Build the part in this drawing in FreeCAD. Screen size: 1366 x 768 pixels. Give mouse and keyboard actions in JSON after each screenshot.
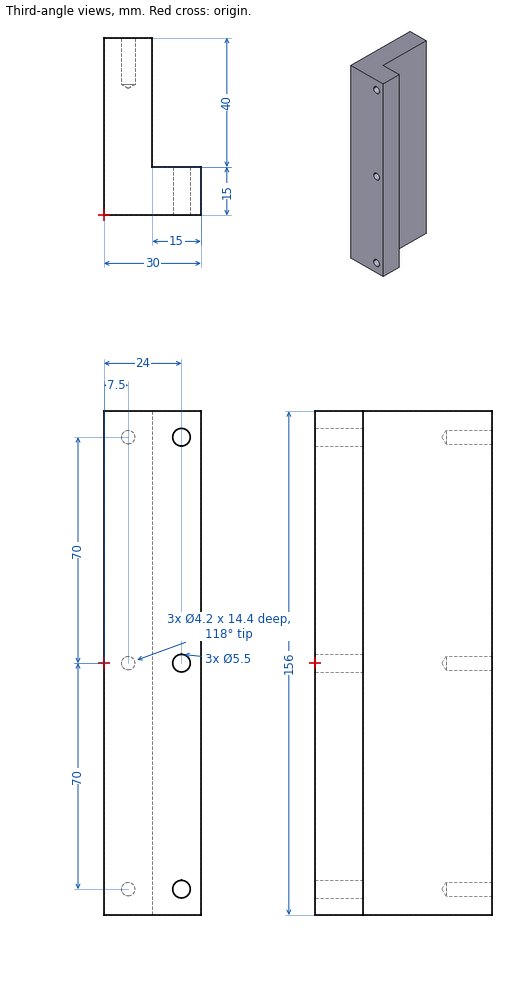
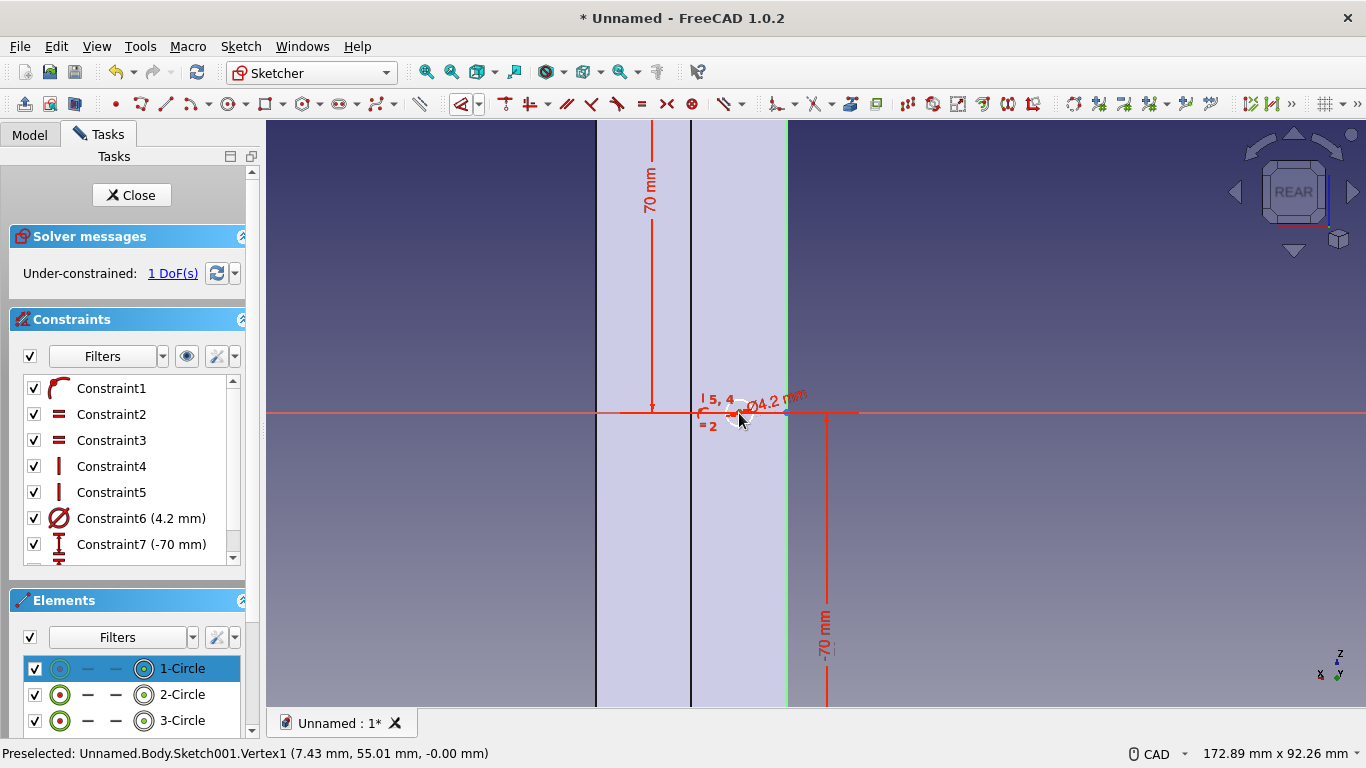
{"action": "key", "text": "l"}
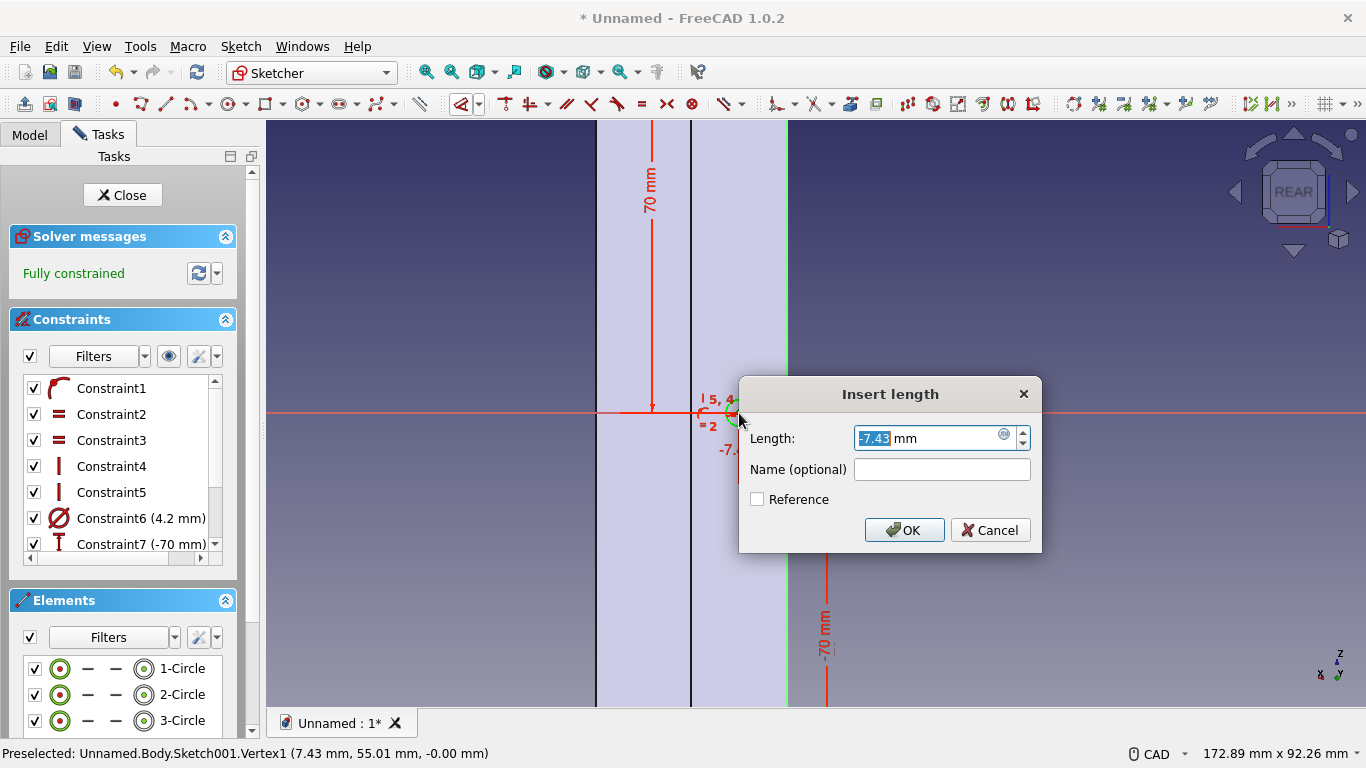
{"action": "type", "text": "-7.5"}
{"action": "key", "text": "Return"}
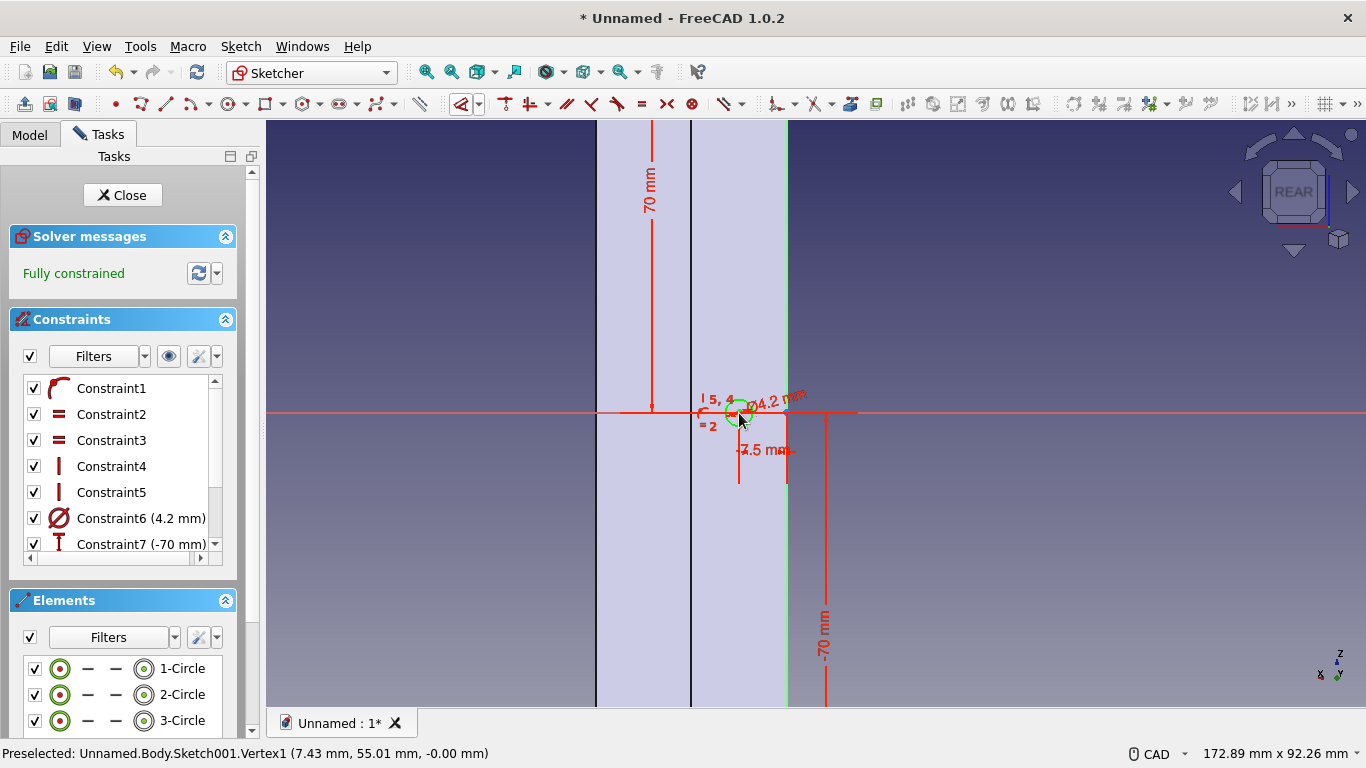
{"action": "left_click", "coordinate": [123, 195]}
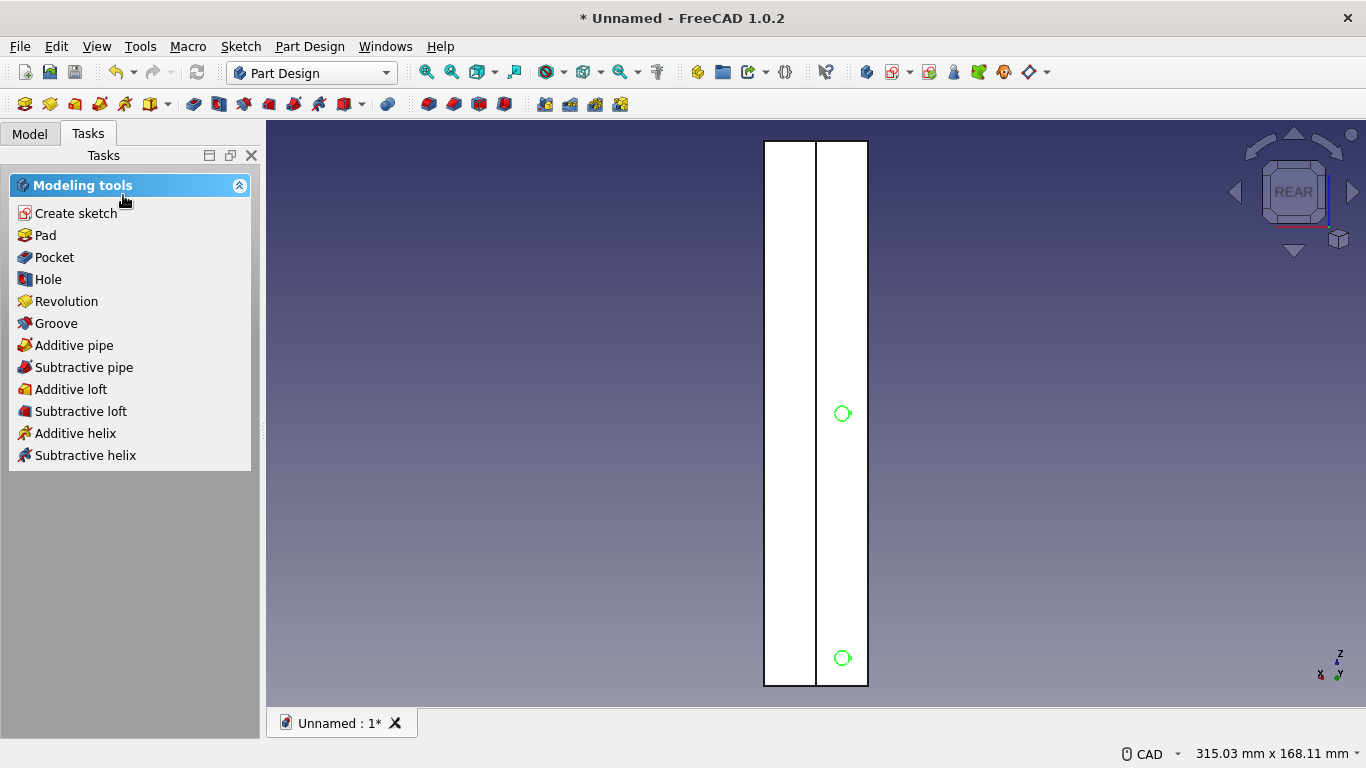
{"action": "left_click", "coordinate": [219, 104]}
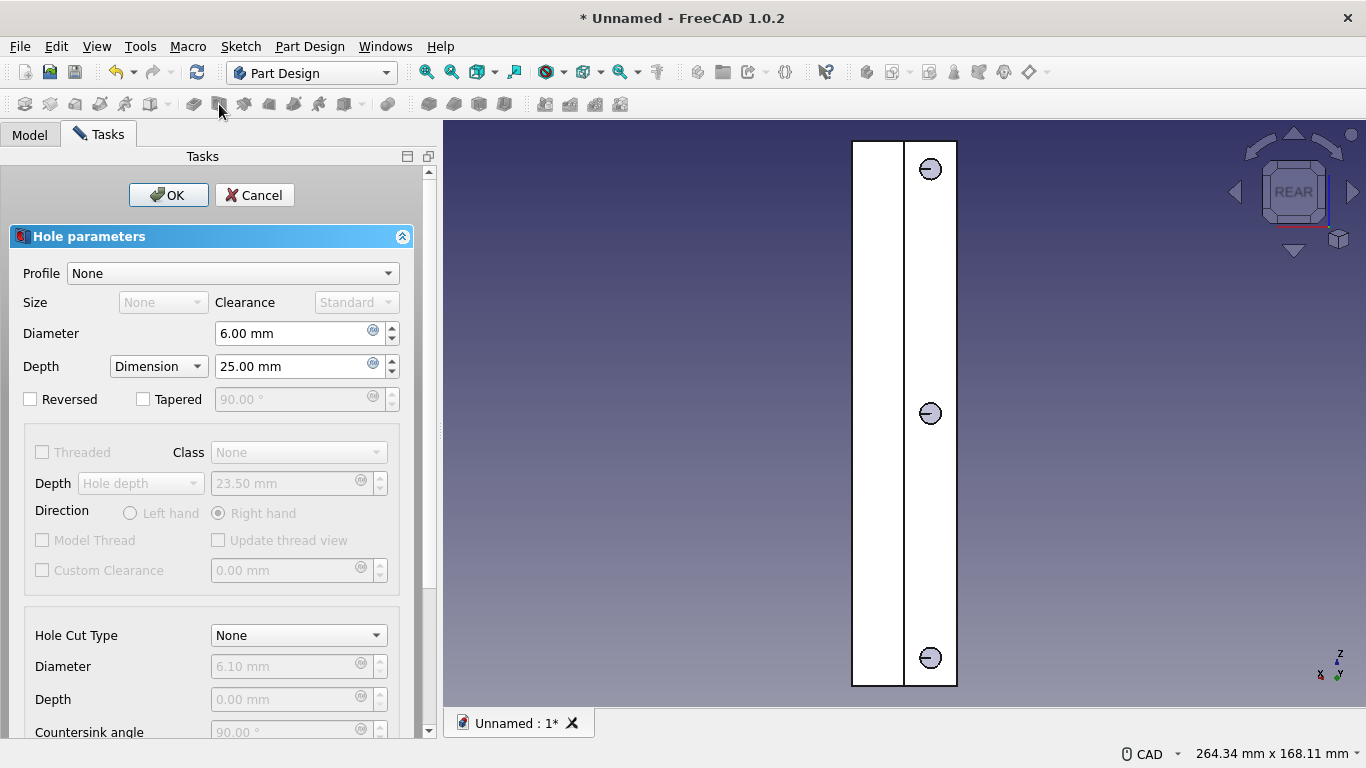
{"action": "triple_click", "coordinate": [300, 334]}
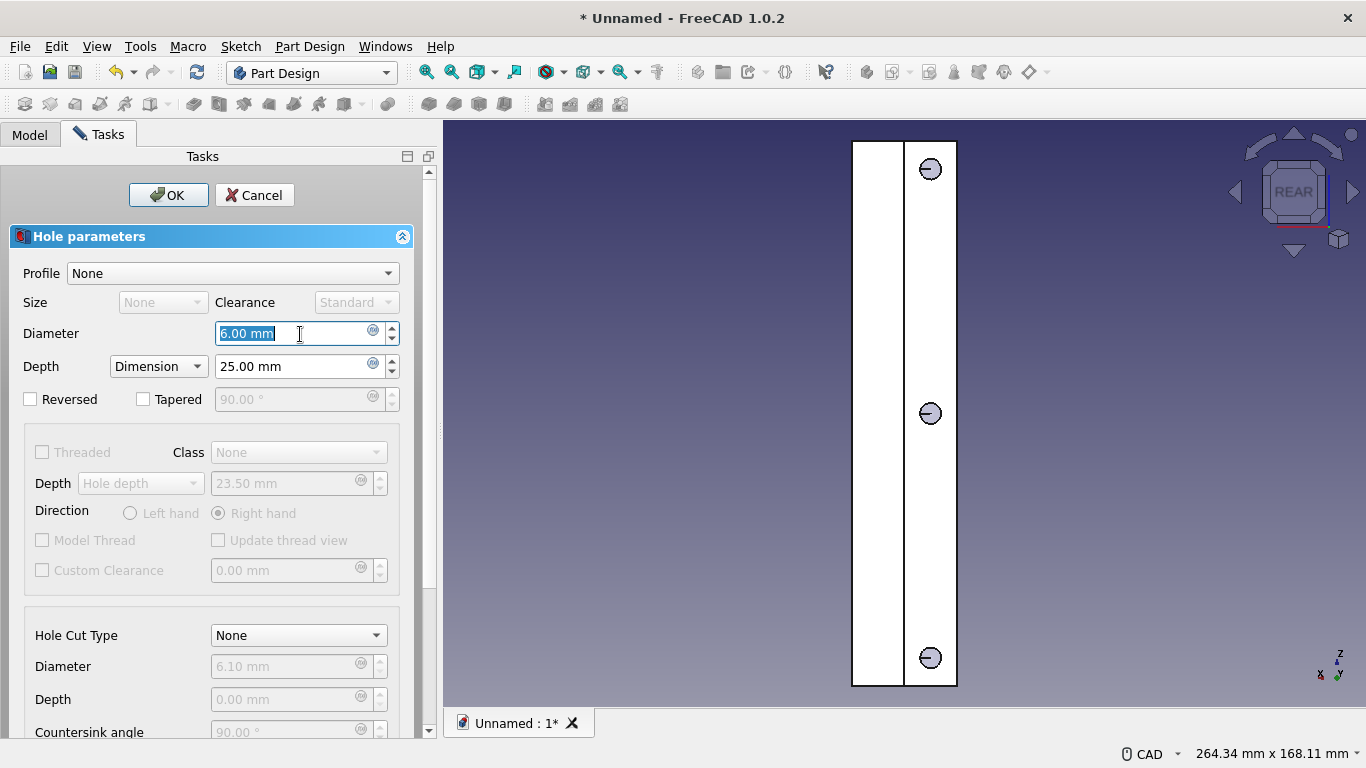
{"action": "type", "text": "4.2"}
{"action": "key", "text": "Tab"}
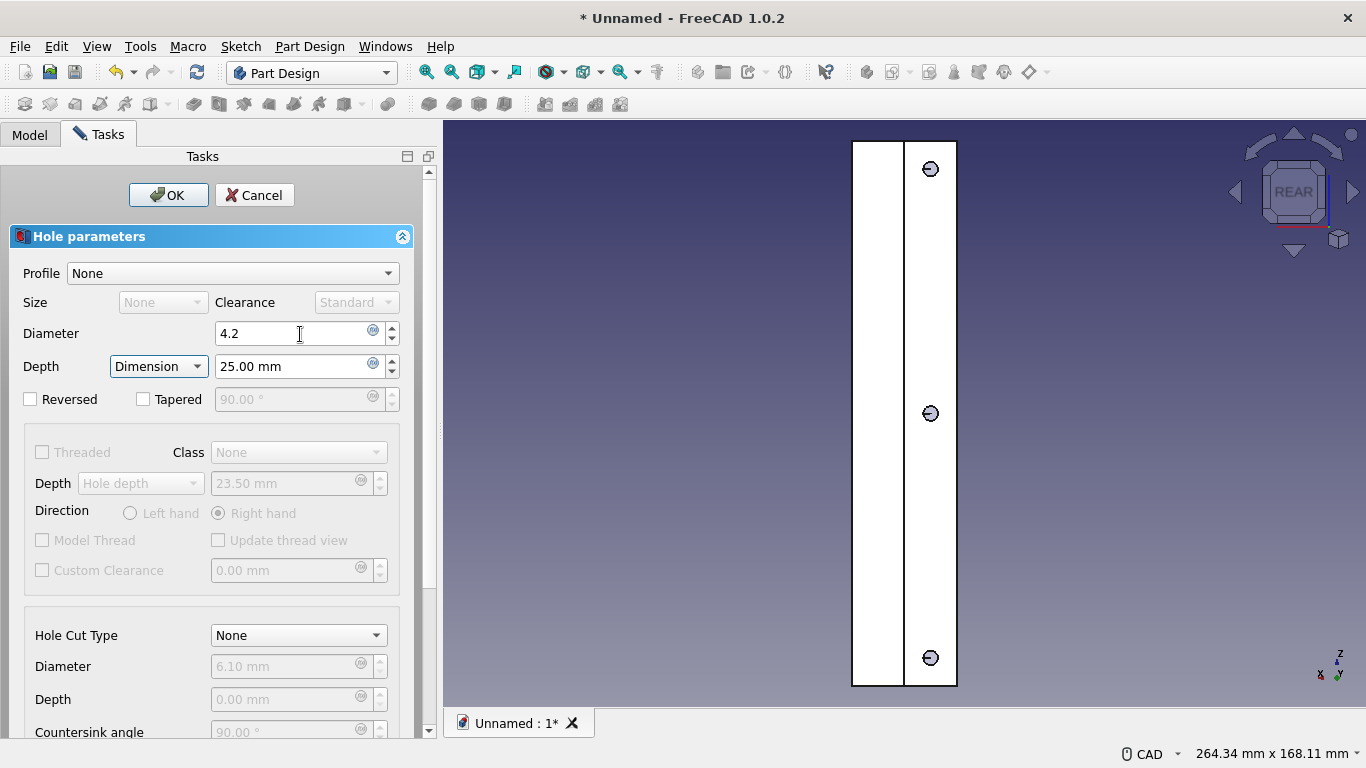
{"action": "triple_click", "coordinate": [300, 366]}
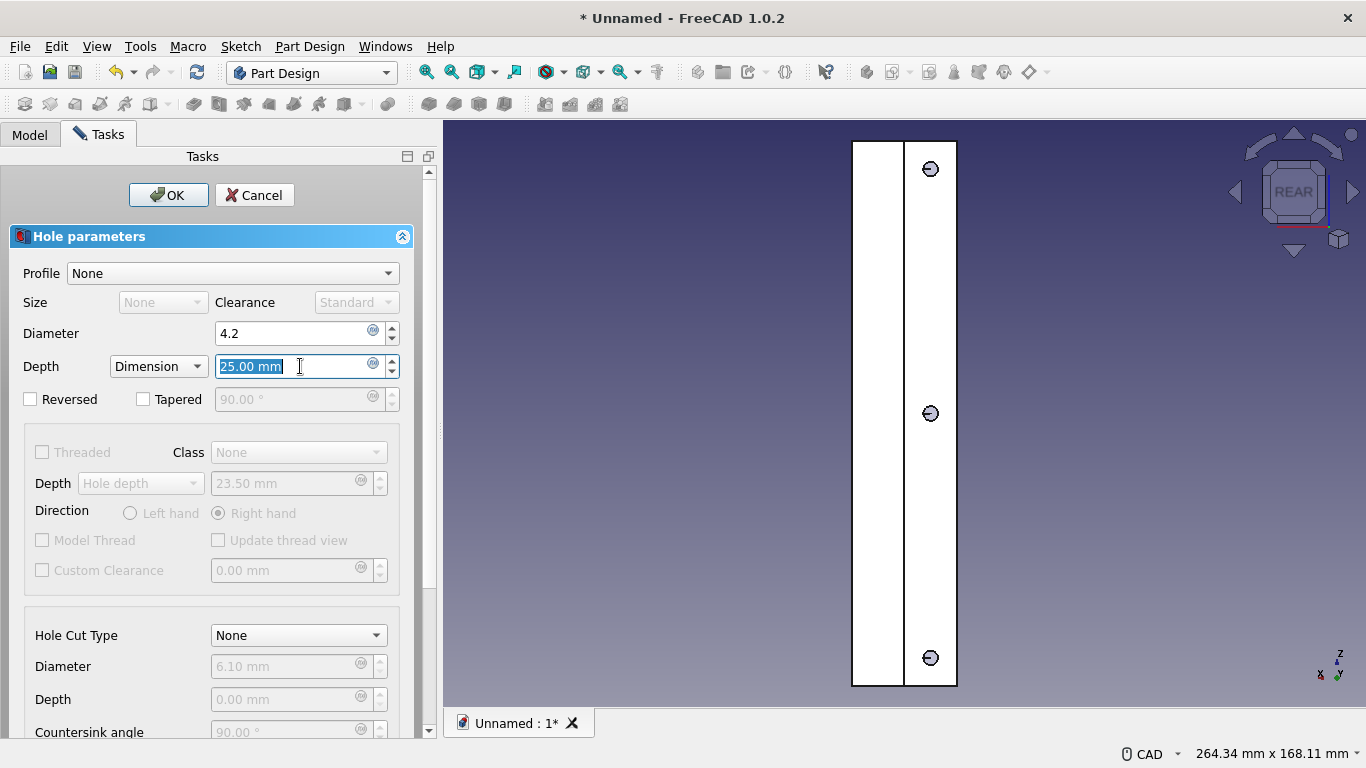
{"action": "type", "text": "14.4"}
{"action": "key", "text": "Tab"}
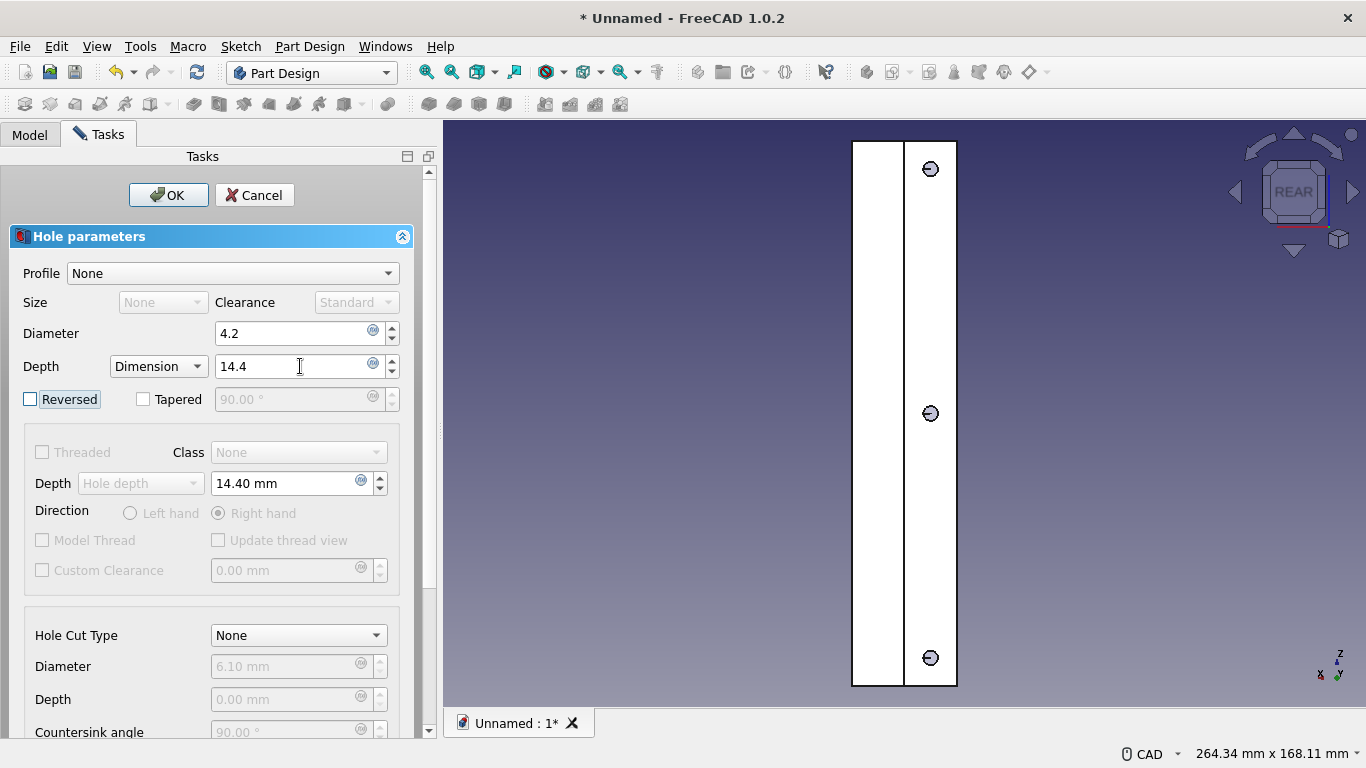
{"action": "left_click", "coordinate": [169, 195]}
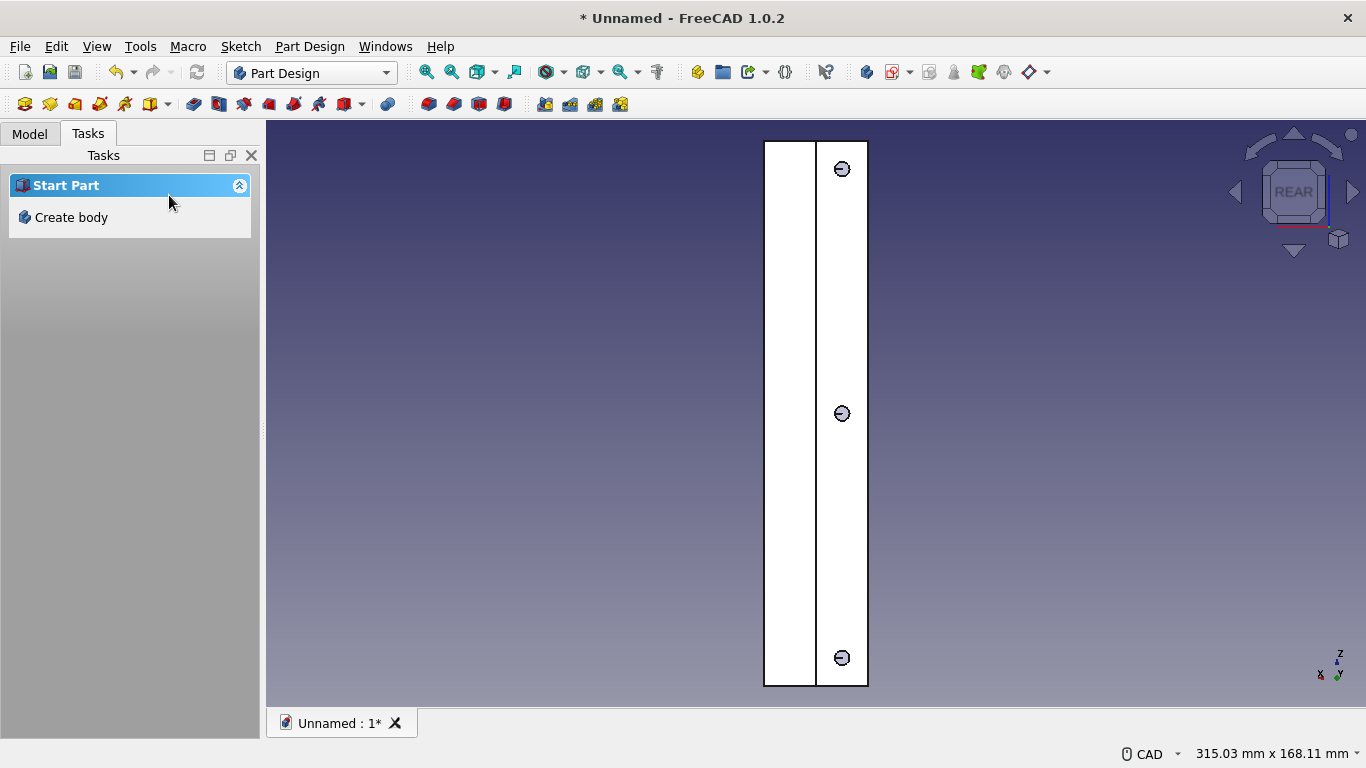
{"action": "left_click", "coordinate": [790, 179]}